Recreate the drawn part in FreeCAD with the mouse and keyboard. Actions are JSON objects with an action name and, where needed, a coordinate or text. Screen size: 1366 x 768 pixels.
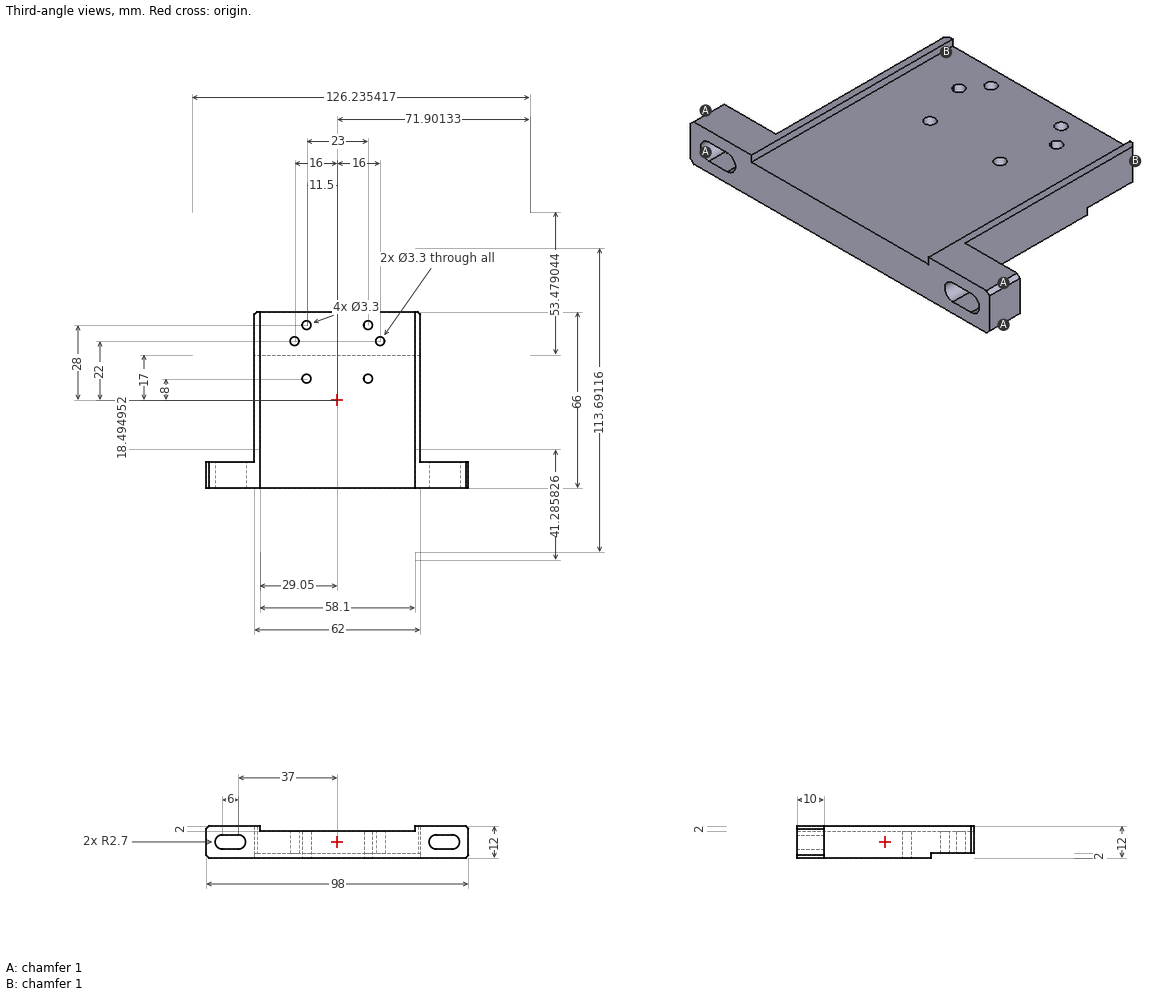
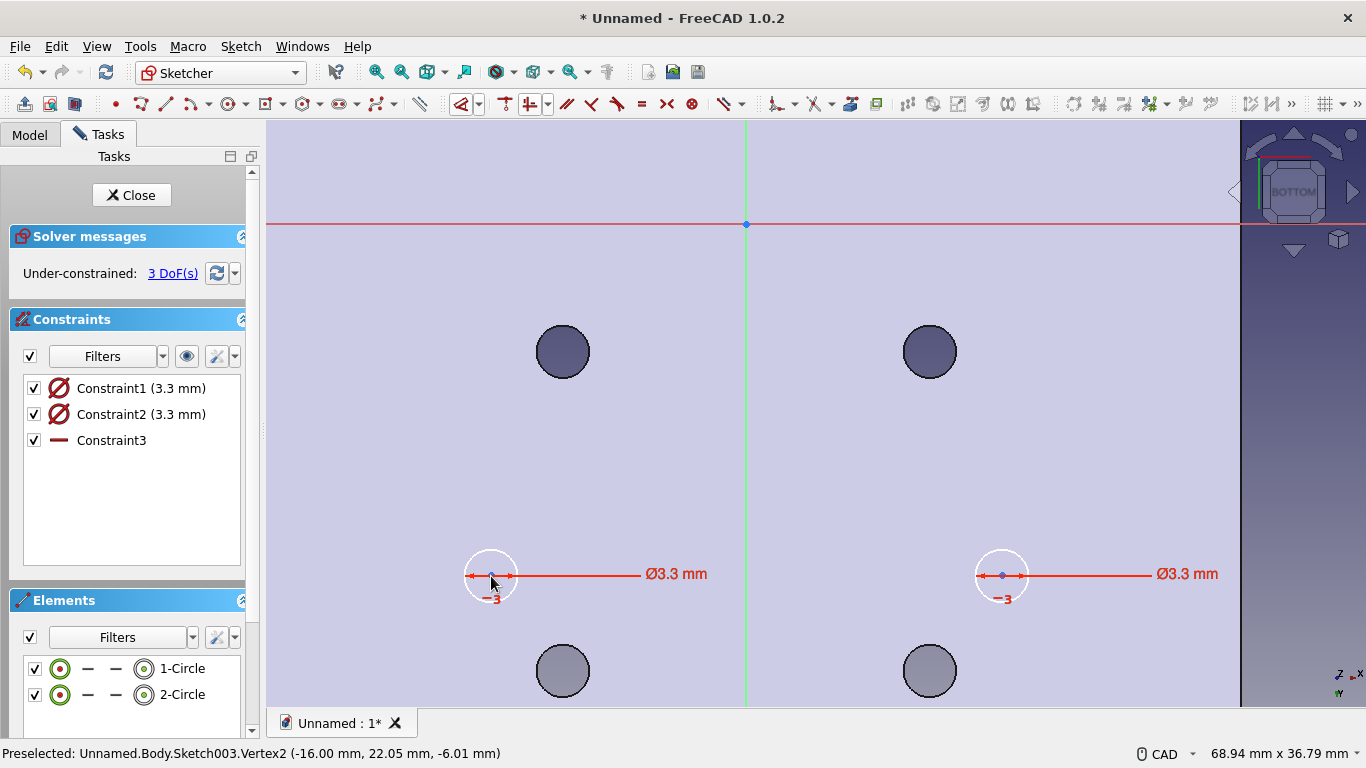
{"action": "left_click", "coordinate": [1002, 576]}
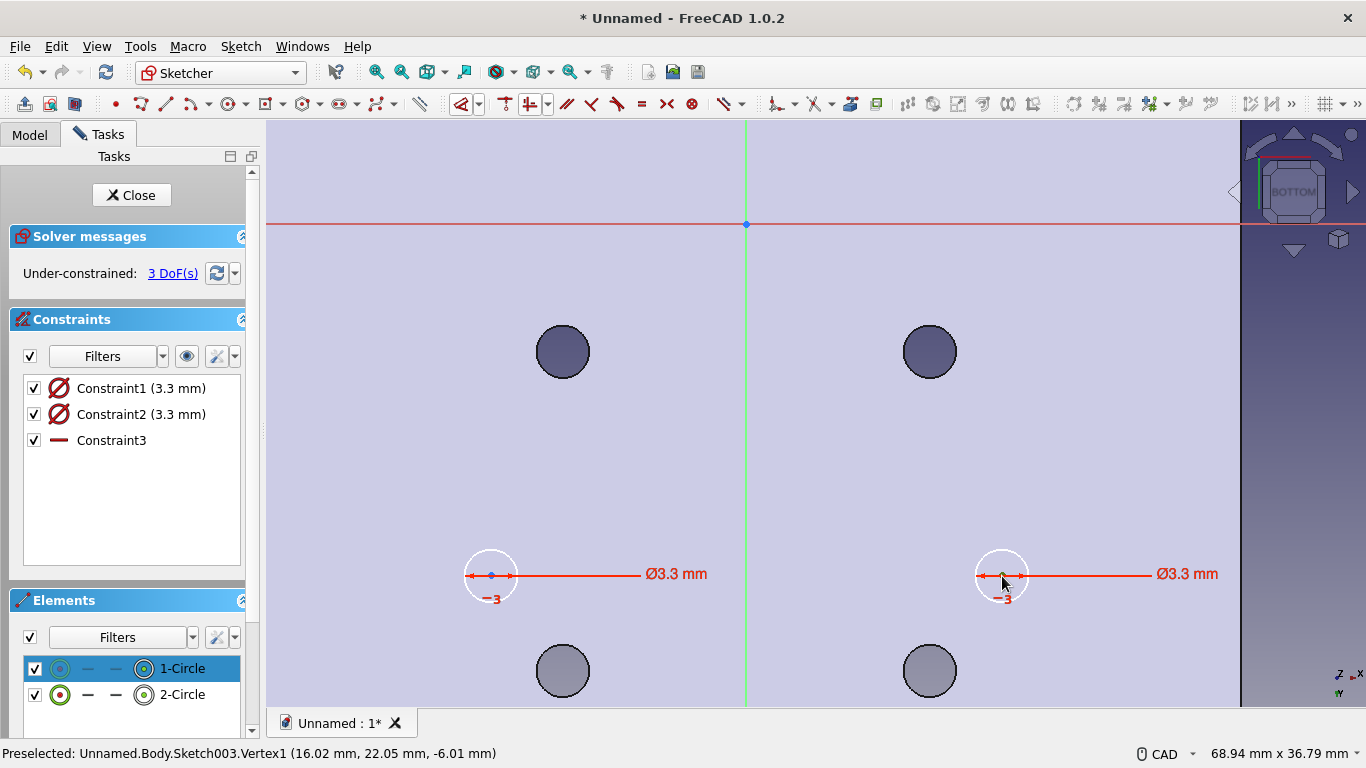
{"action": "left_click", "coordinate": [478, 104]}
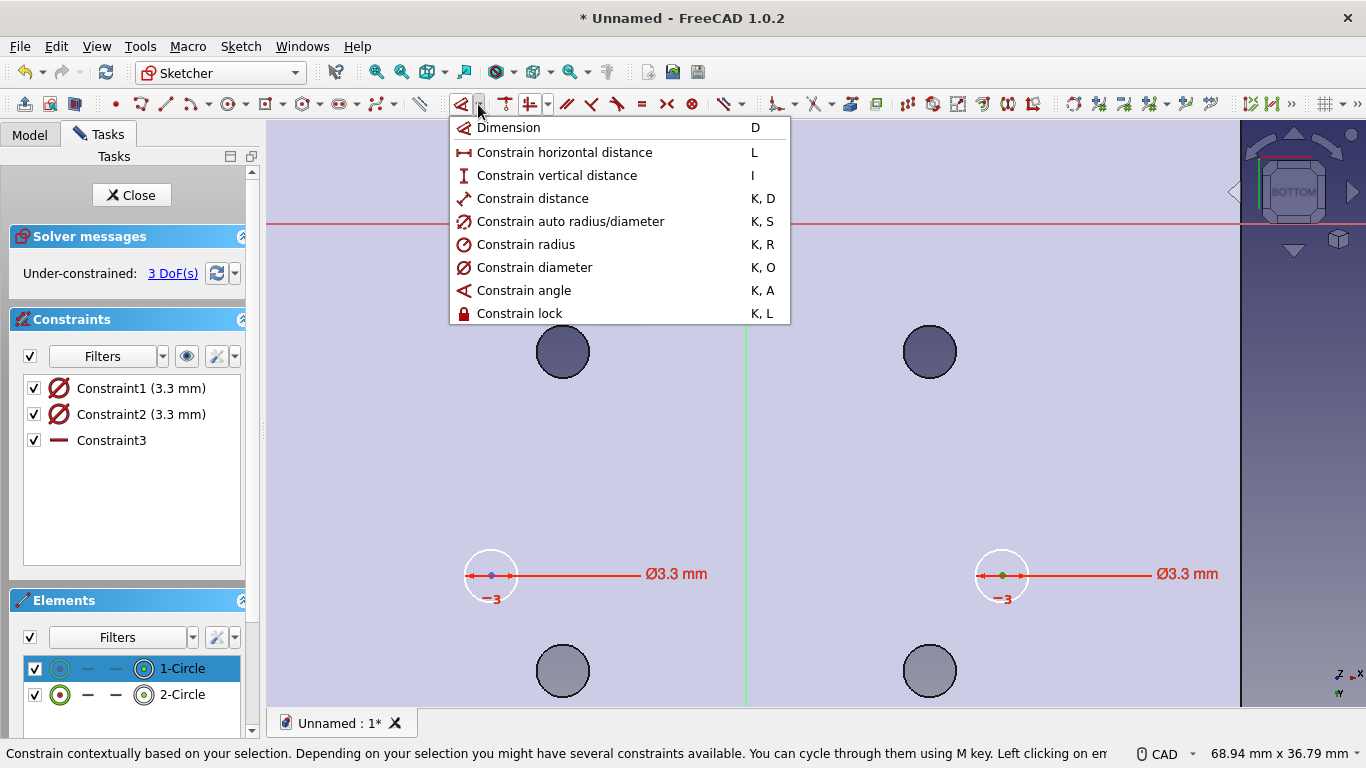
{"action": "left_click", "coordinate": [620, 152]}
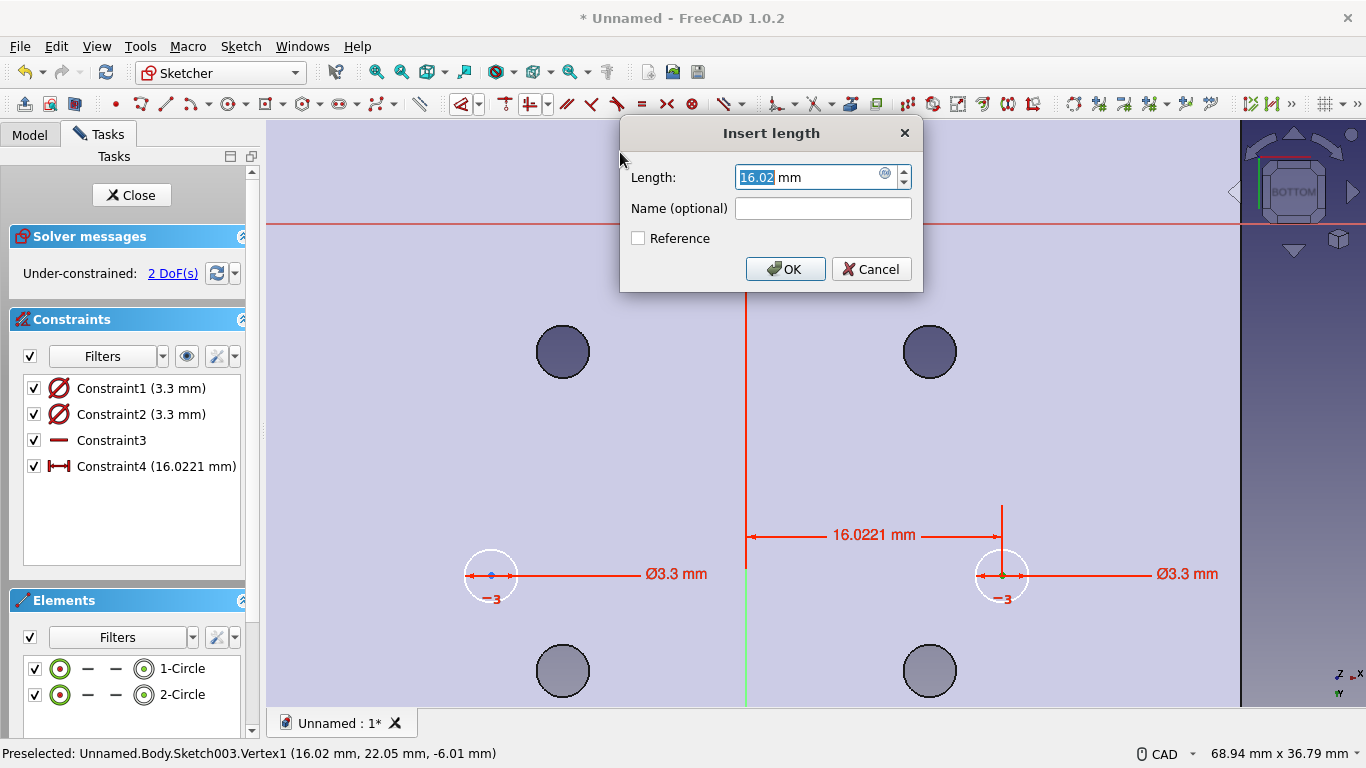
{"action": "type", "text": "16"}
{"action": "key", "text": "Return"}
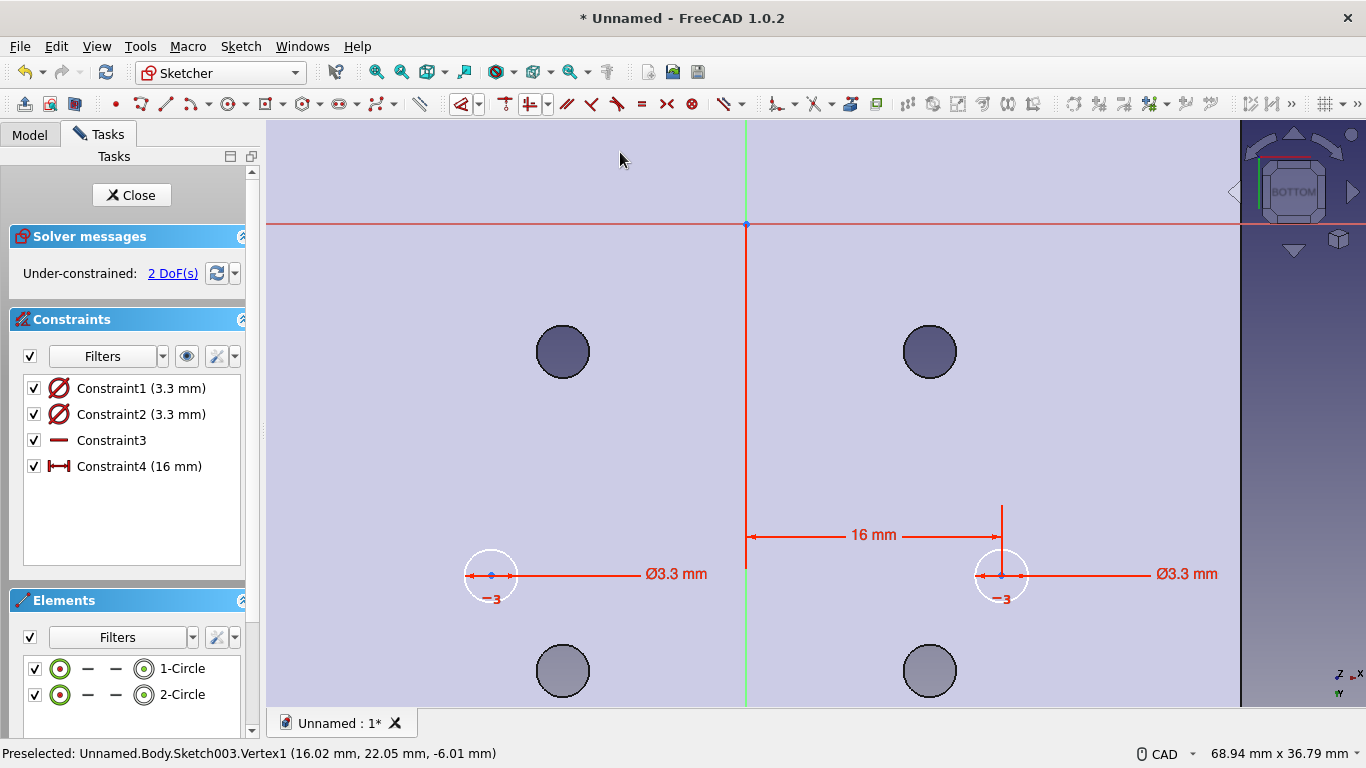
{"action": "left_click", "coordinate": [1002, 576]}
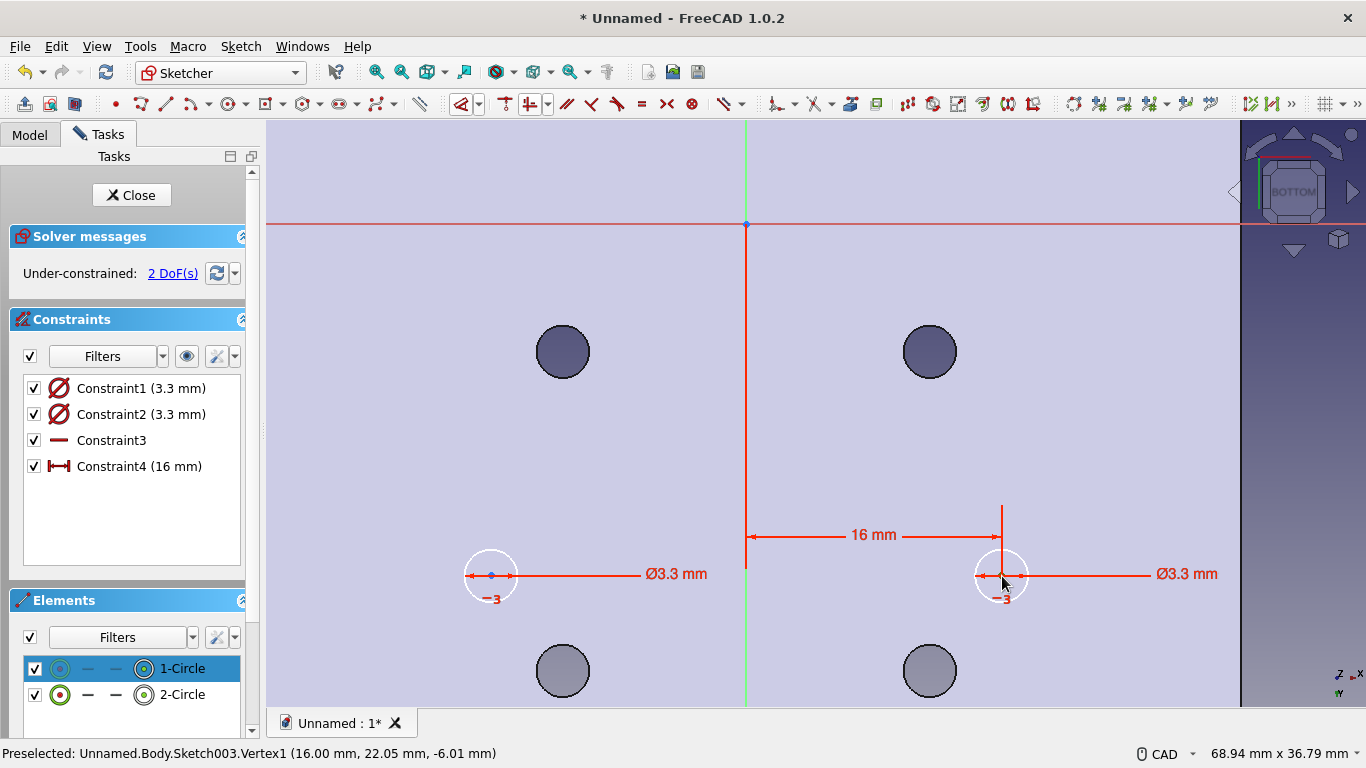
{"action": "left_click", "coordinate": [478, 104]}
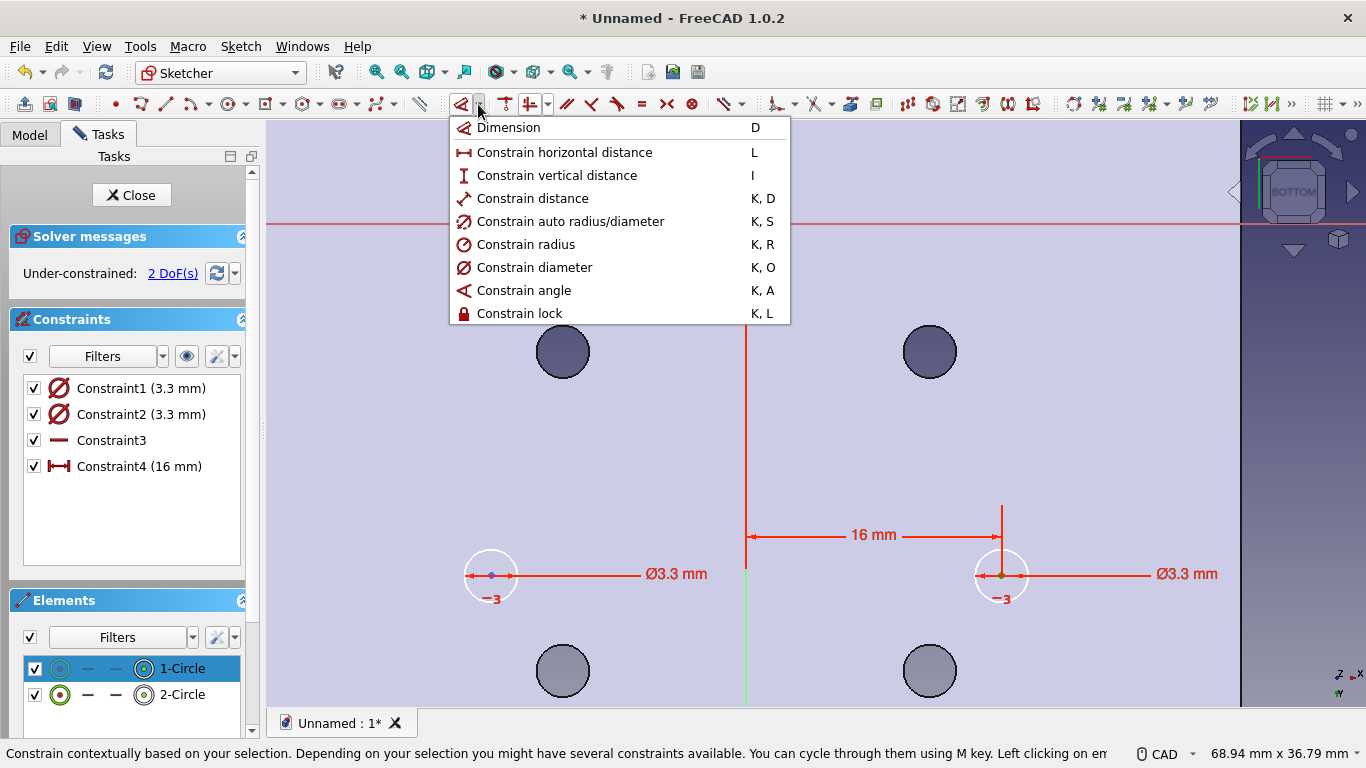
{"action": "left_click", "coordinate": [620, 176]}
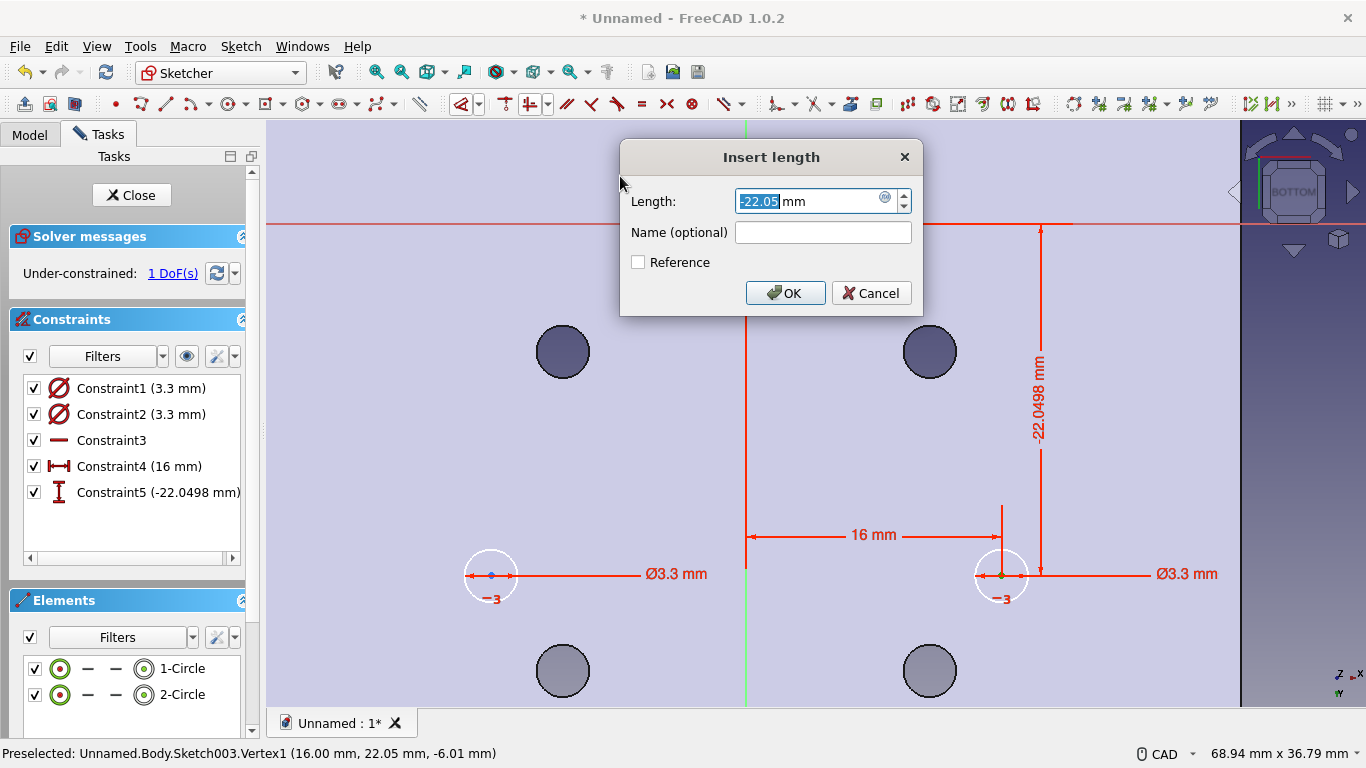
{"action": "type", "text": "-22"}
{"action": "key", "text": "Return"}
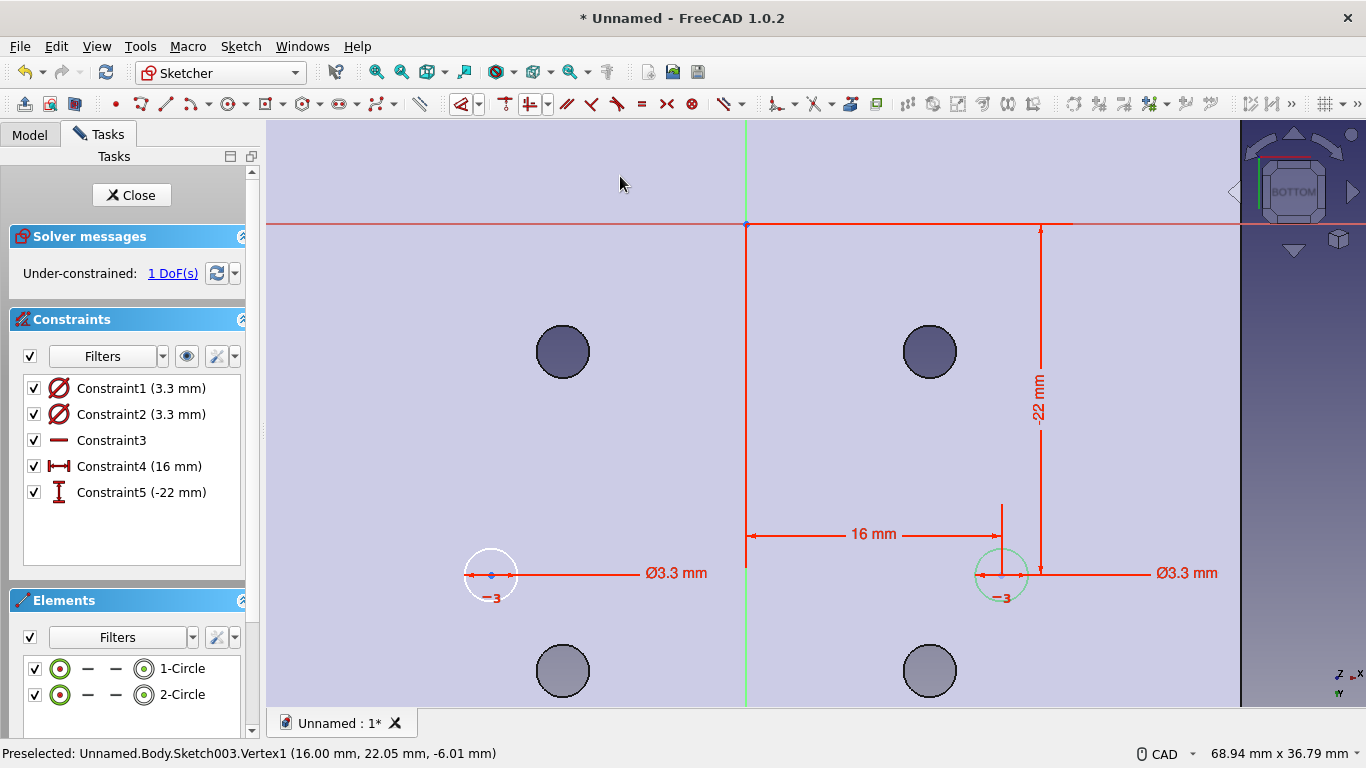
{"action": "left_click", "coordinate": [491, 575]}